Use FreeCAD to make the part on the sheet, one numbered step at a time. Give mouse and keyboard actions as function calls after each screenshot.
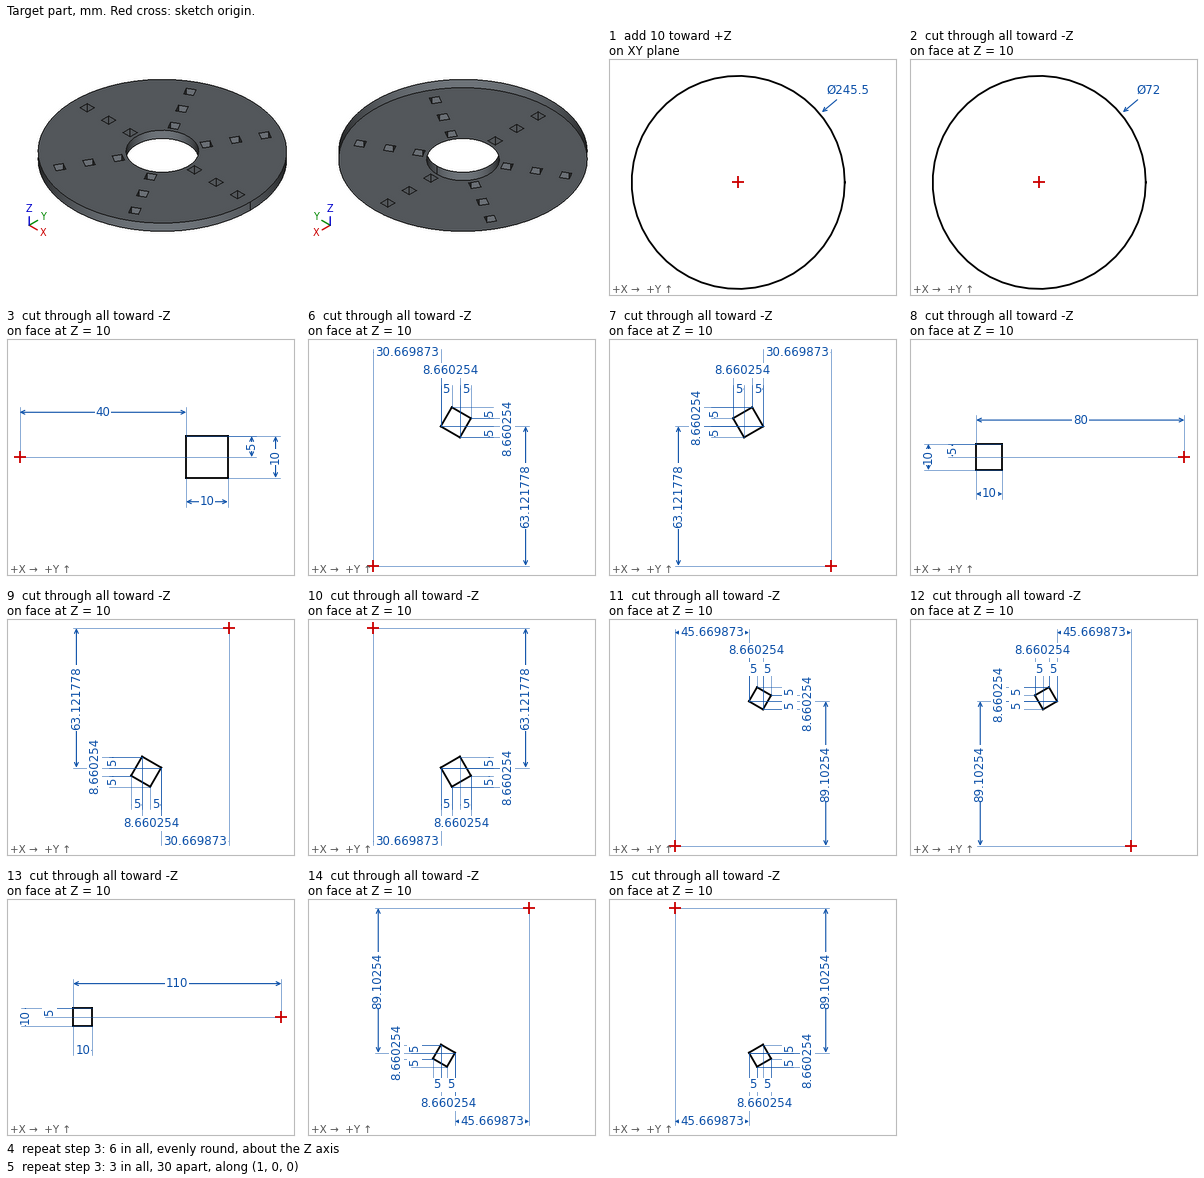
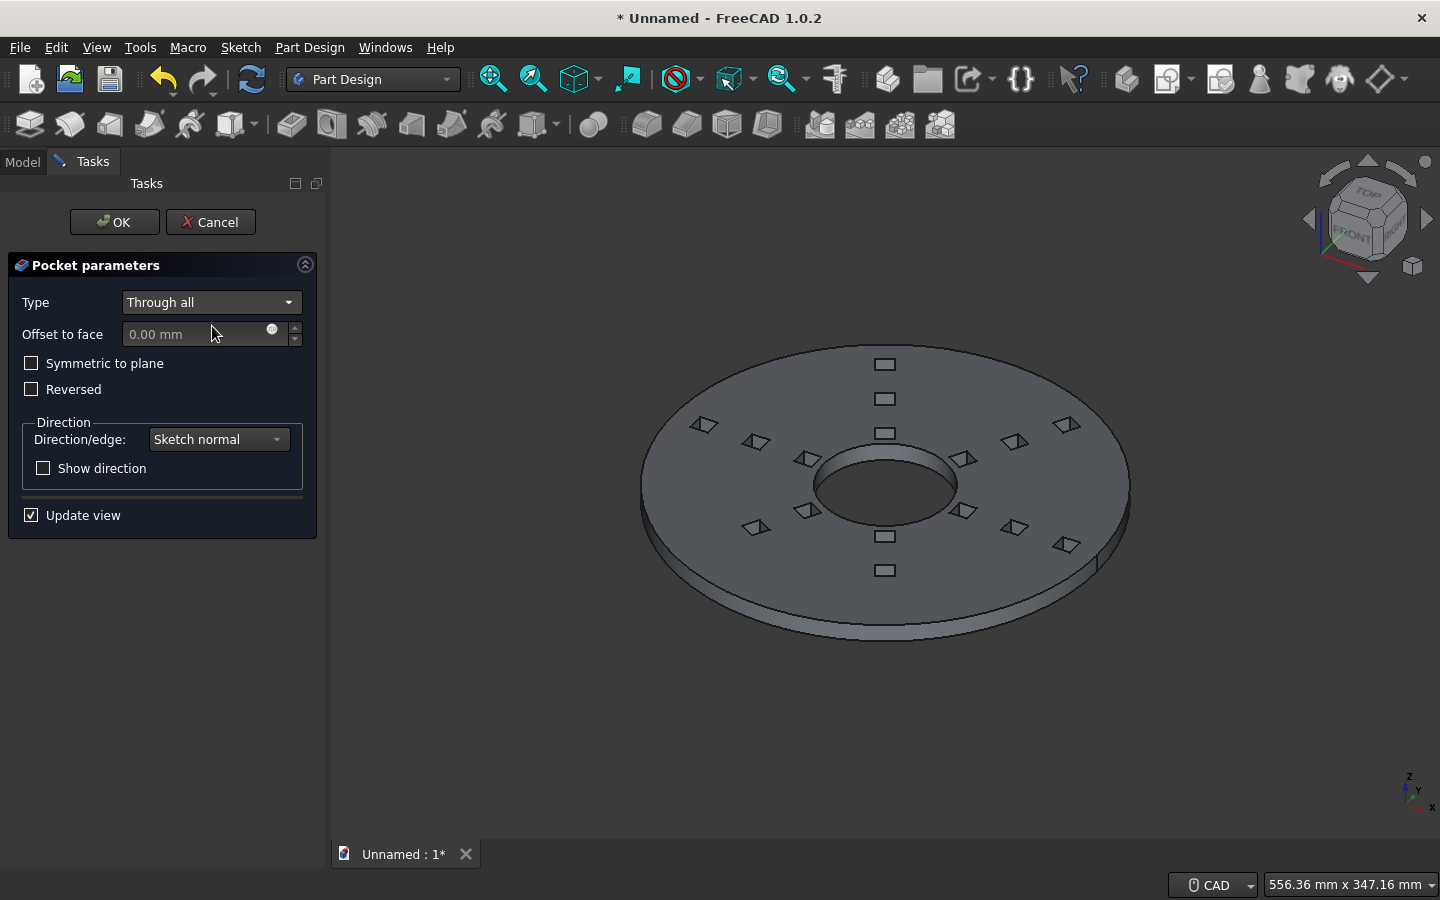
click(115, 222)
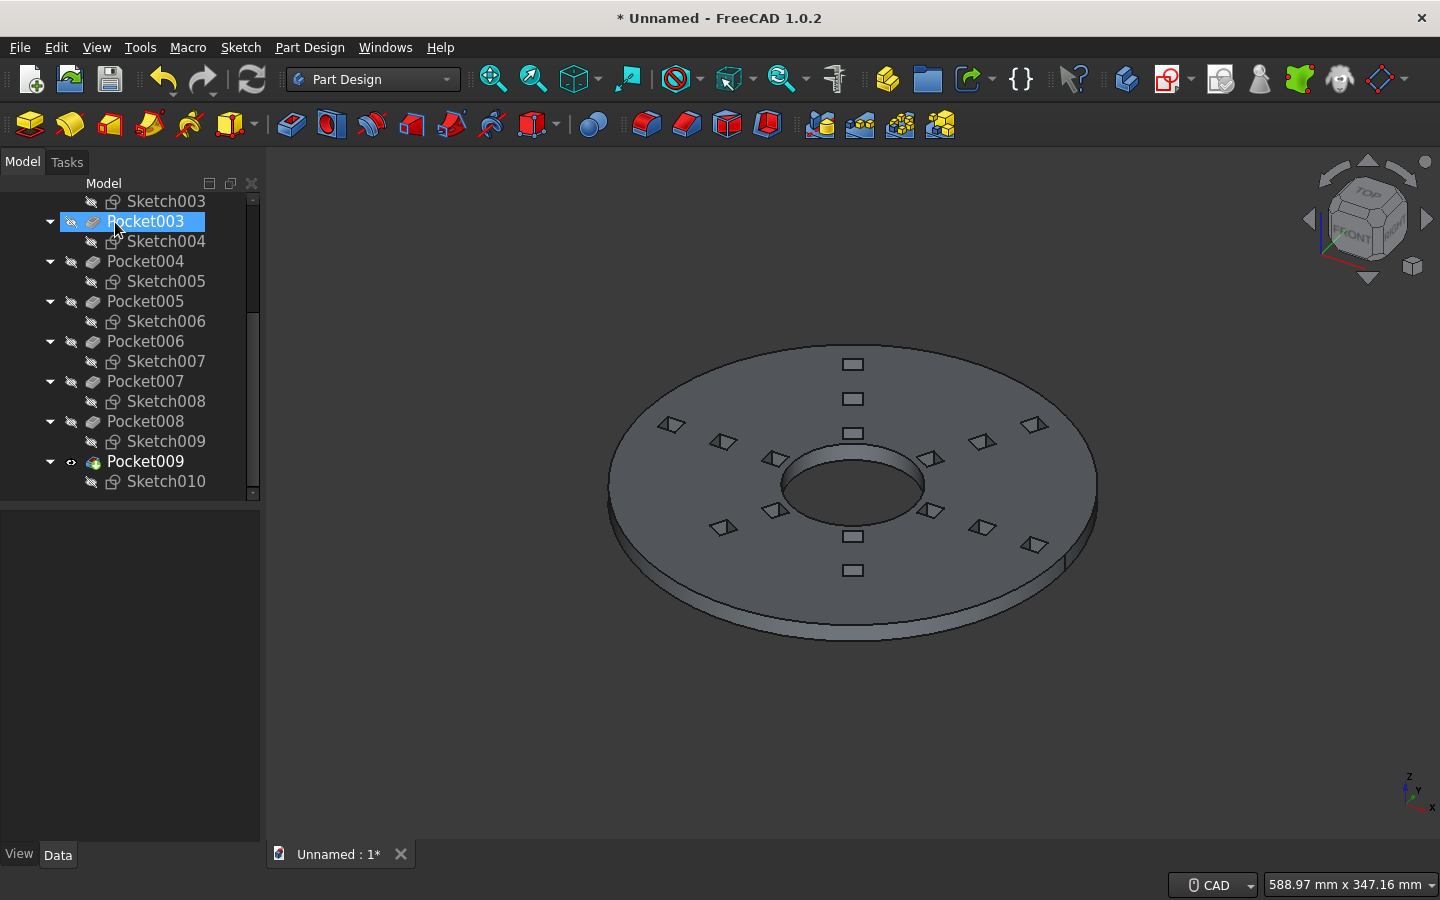
click(923, 414)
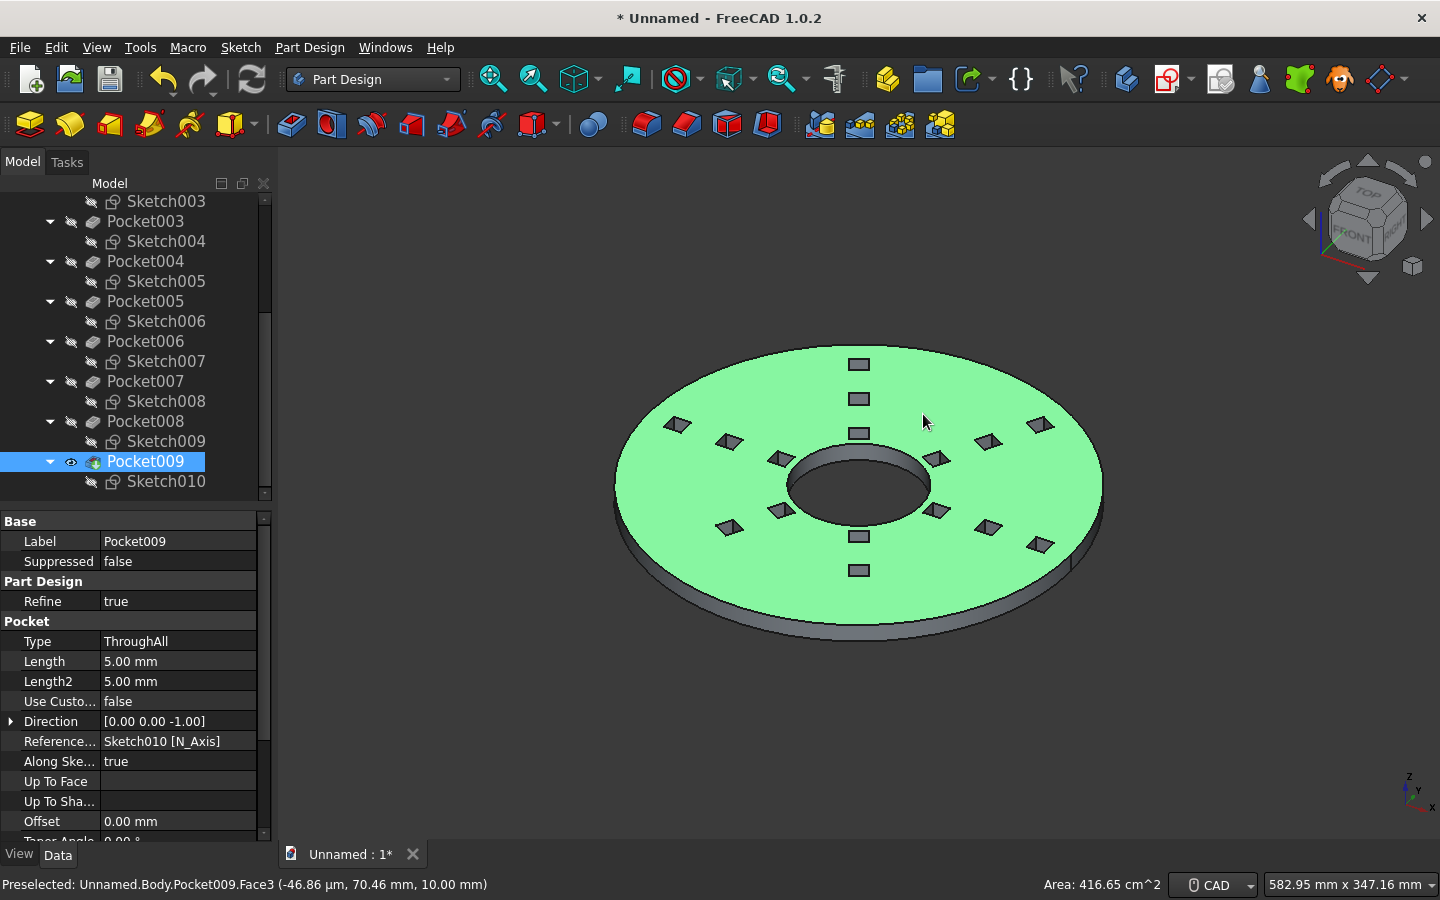
click(1168, 80)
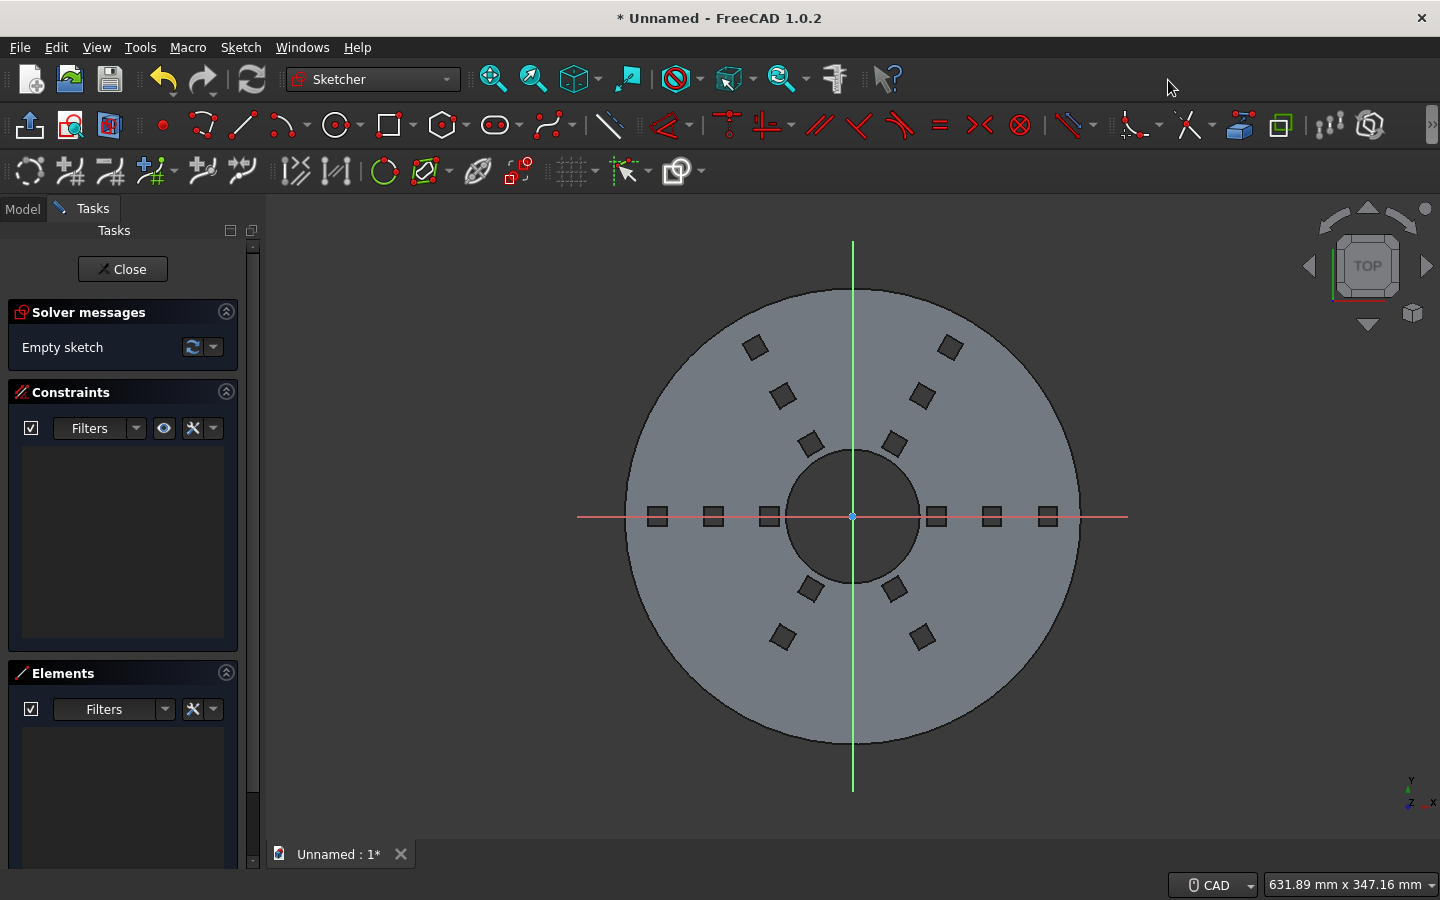
scroll(753, 696, up, 14)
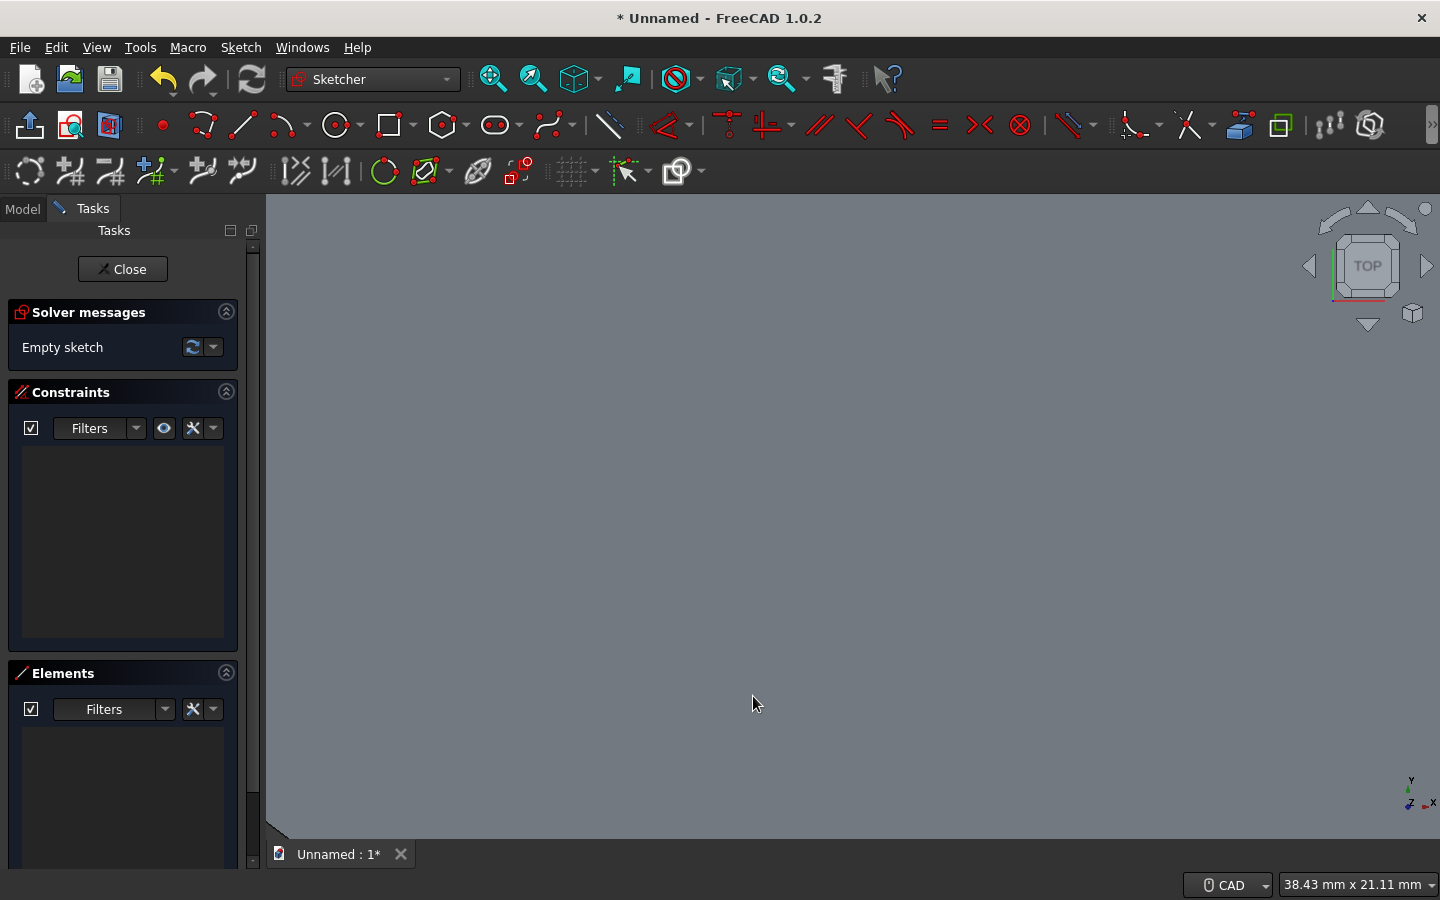
click(204, 126)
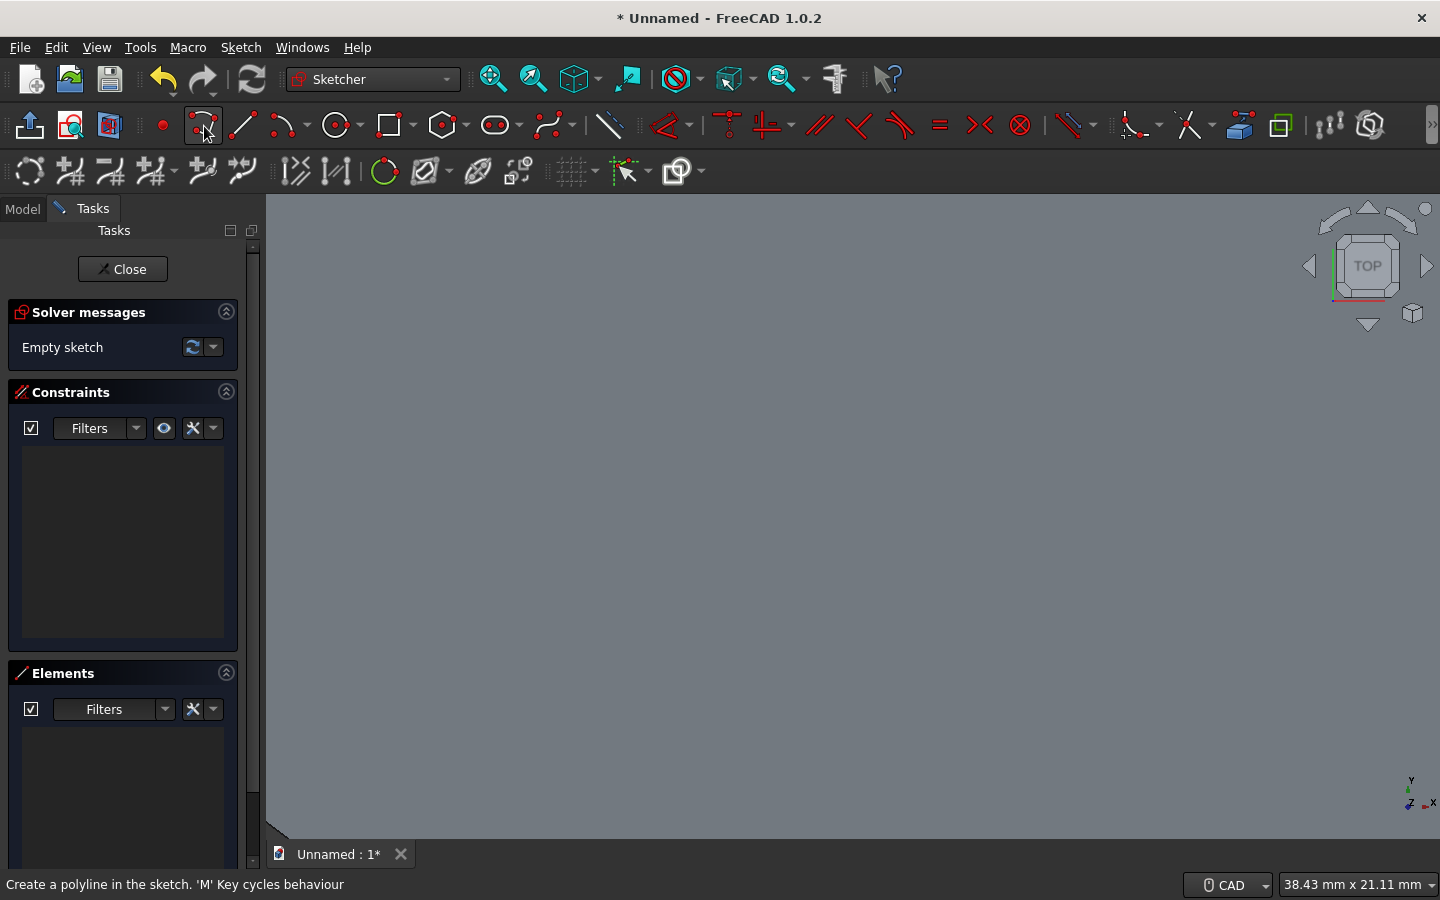
click(993, 454)
click(729, 302)
click(576, 566)
click(840, 719)
click(993, 455)
key(Escape)
key(Escape)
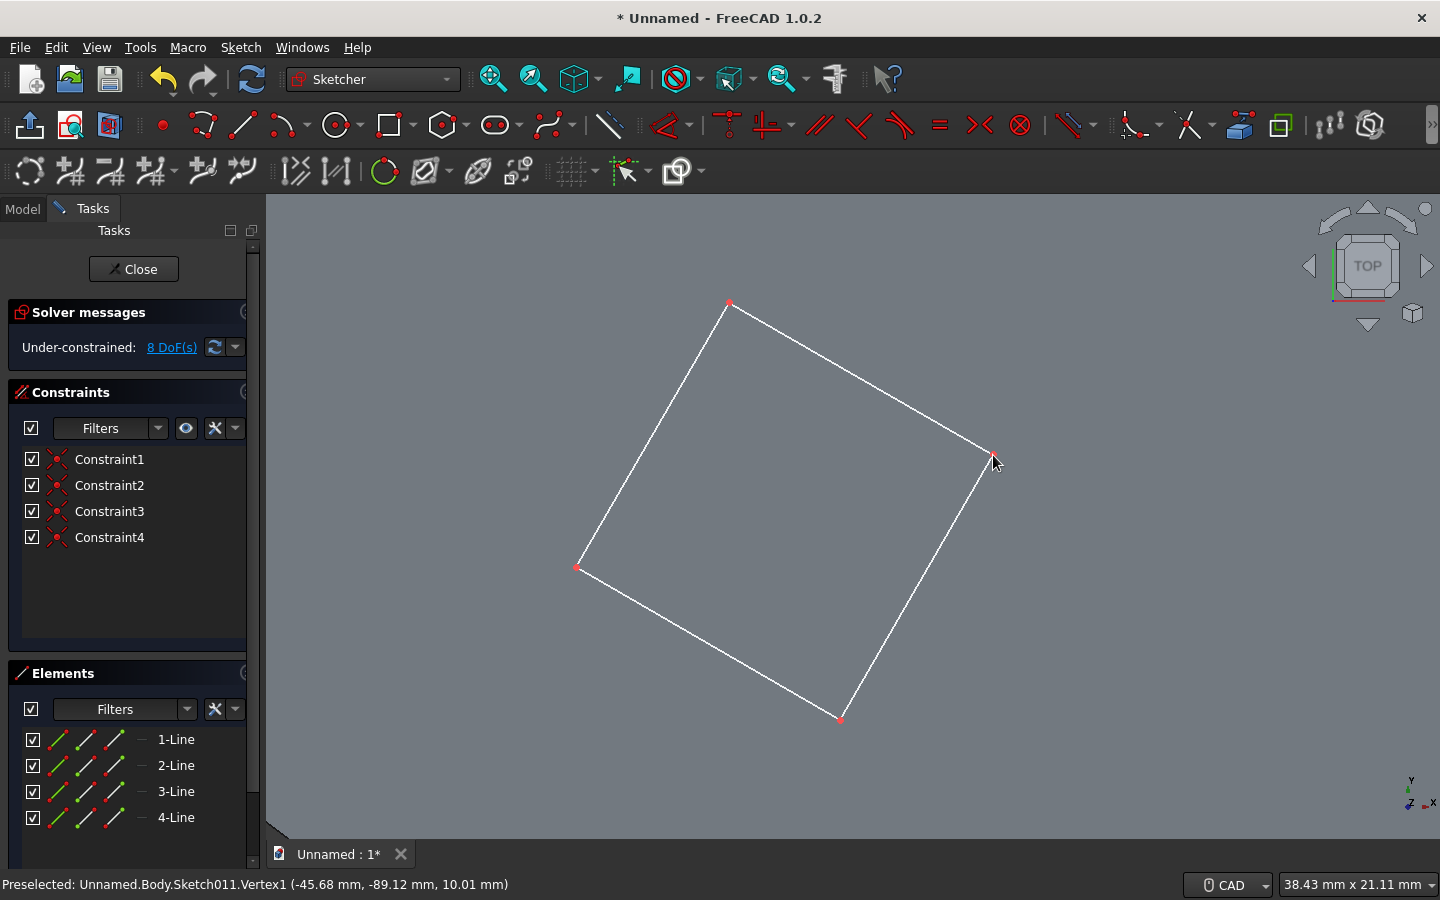
click(664, 126)